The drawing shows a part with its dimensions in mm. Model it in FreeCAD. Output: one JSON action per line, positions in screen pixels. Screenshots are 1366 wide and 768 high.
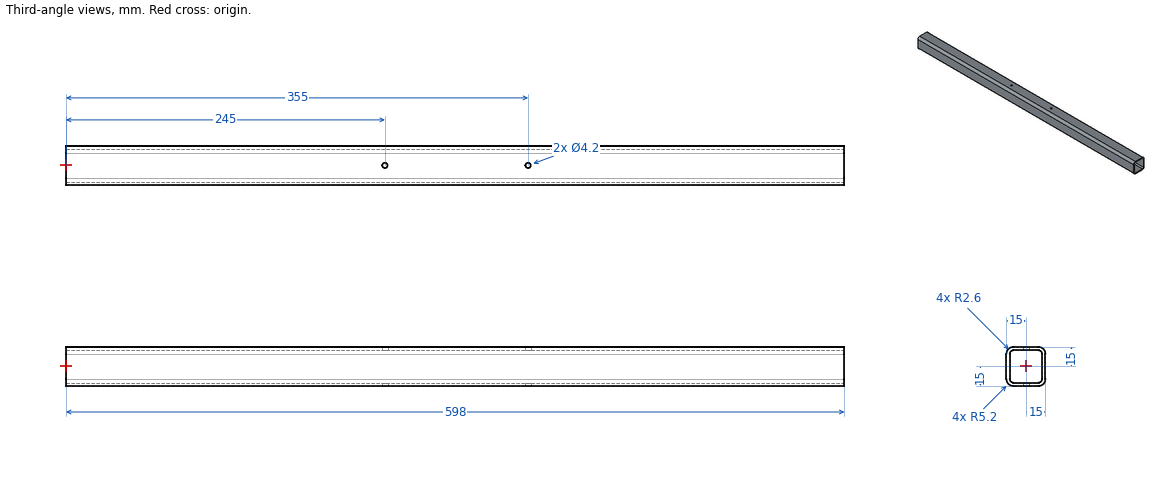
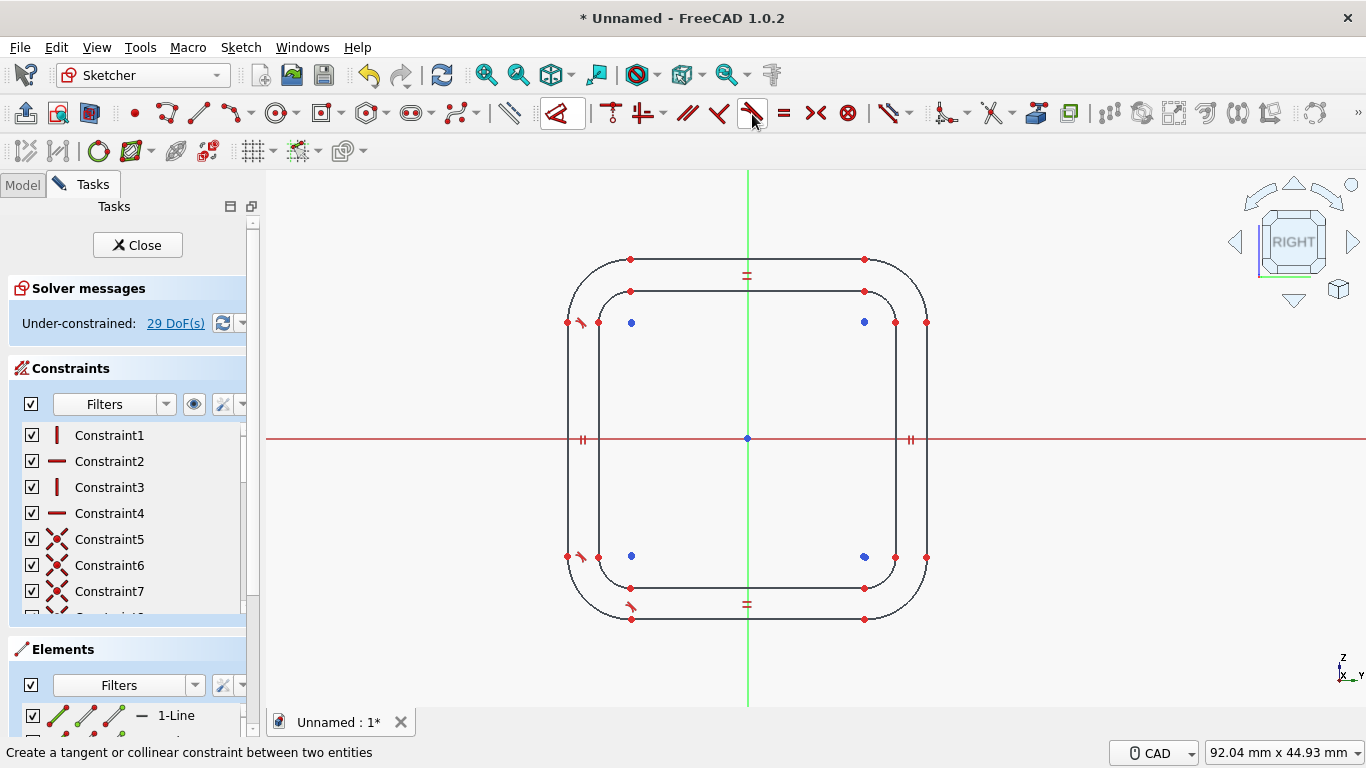
{"action": "left_click", "coordinate": [701, 619]}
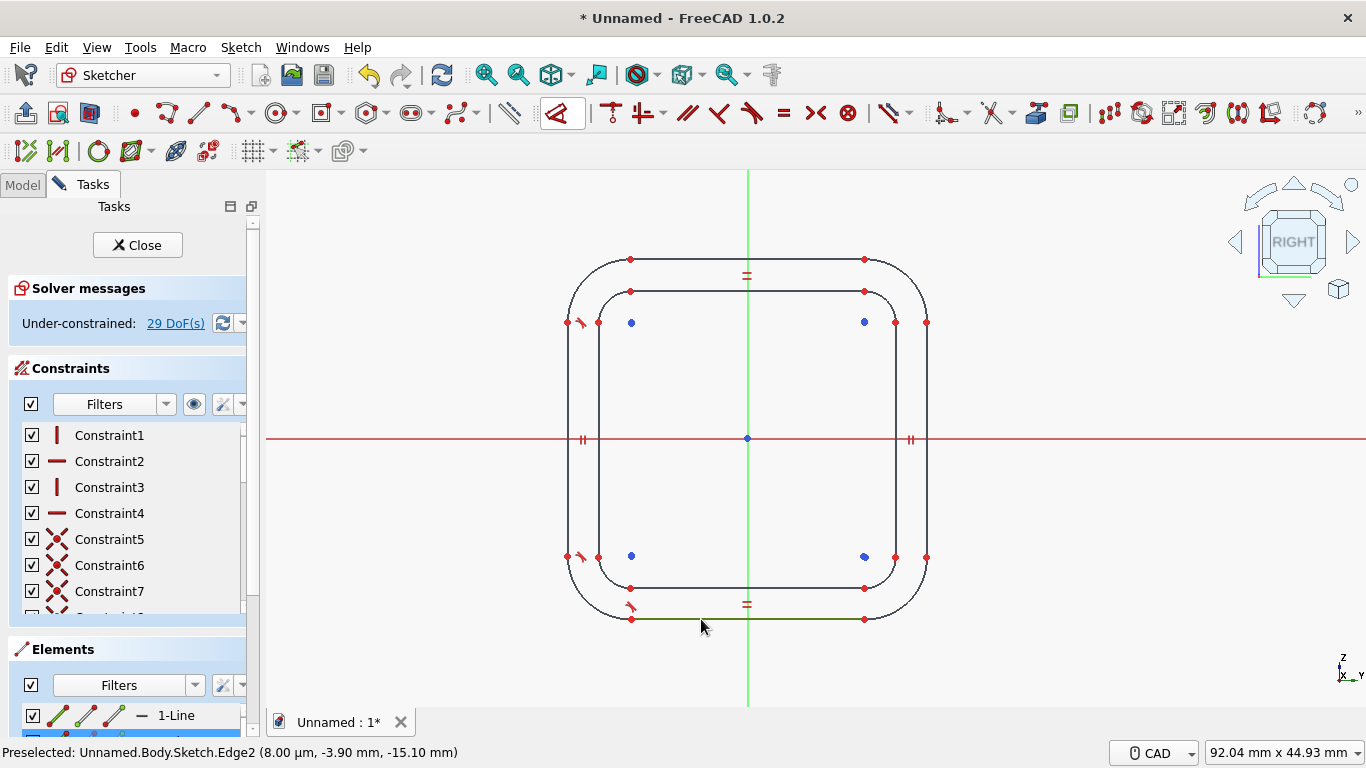
{"action": "left_click", "coordinate": [893, 613]}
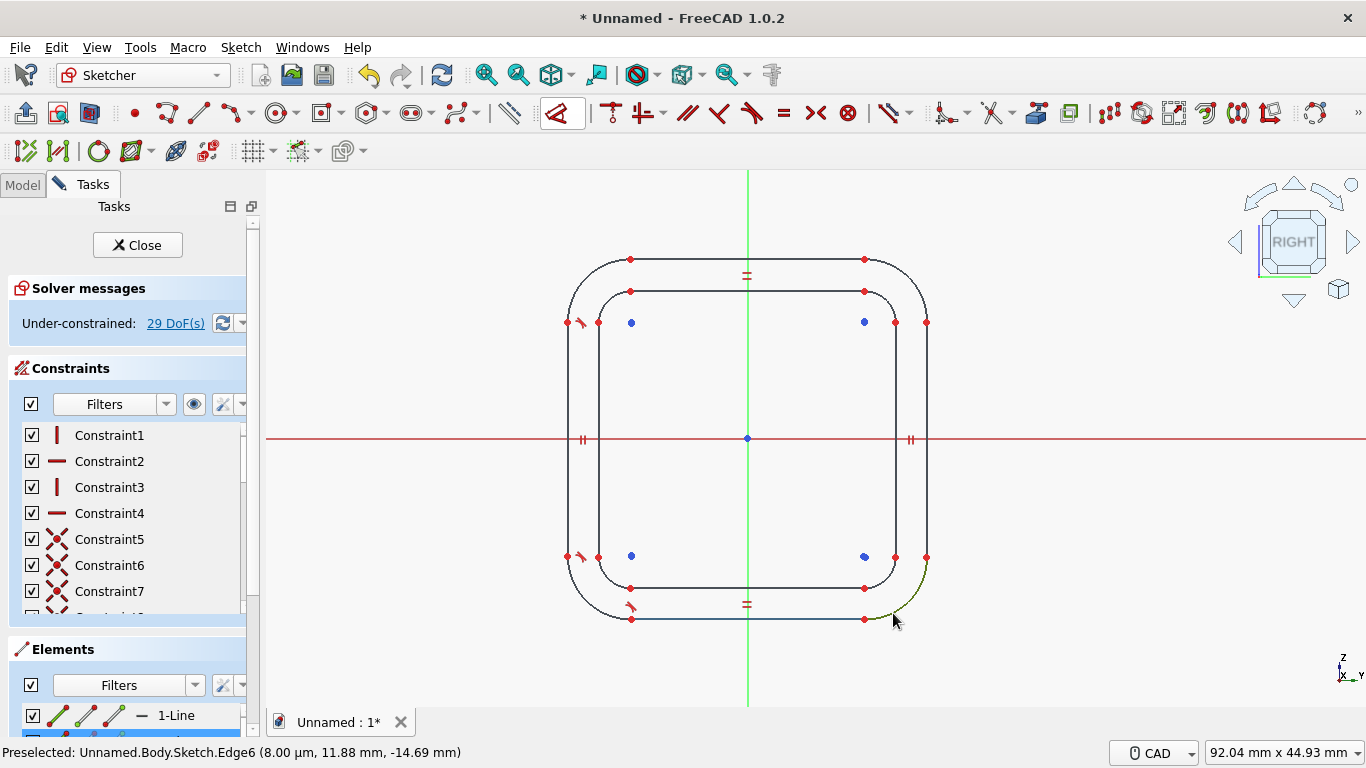
{"action": "left_click", "coordinate": [752, 114]}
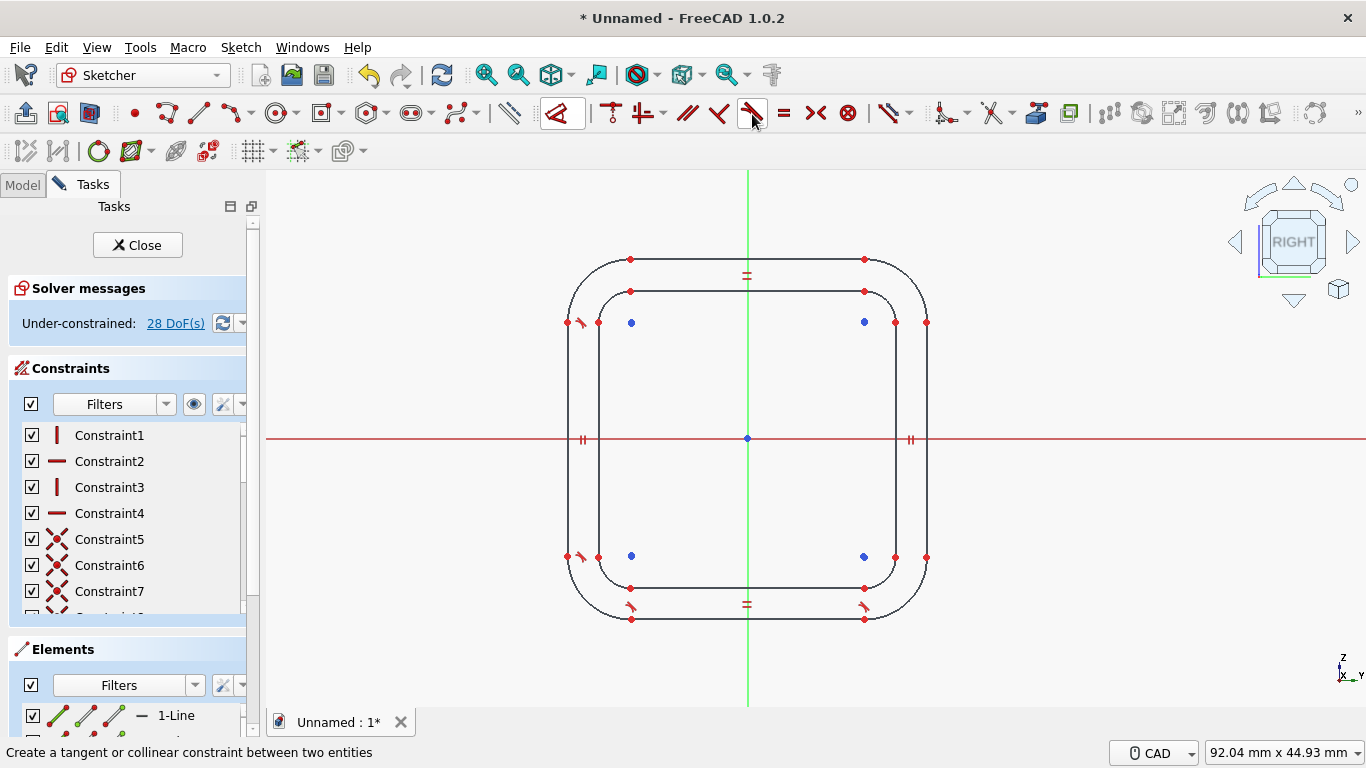
{"action": "left_click", "coordinate": [927, 487]}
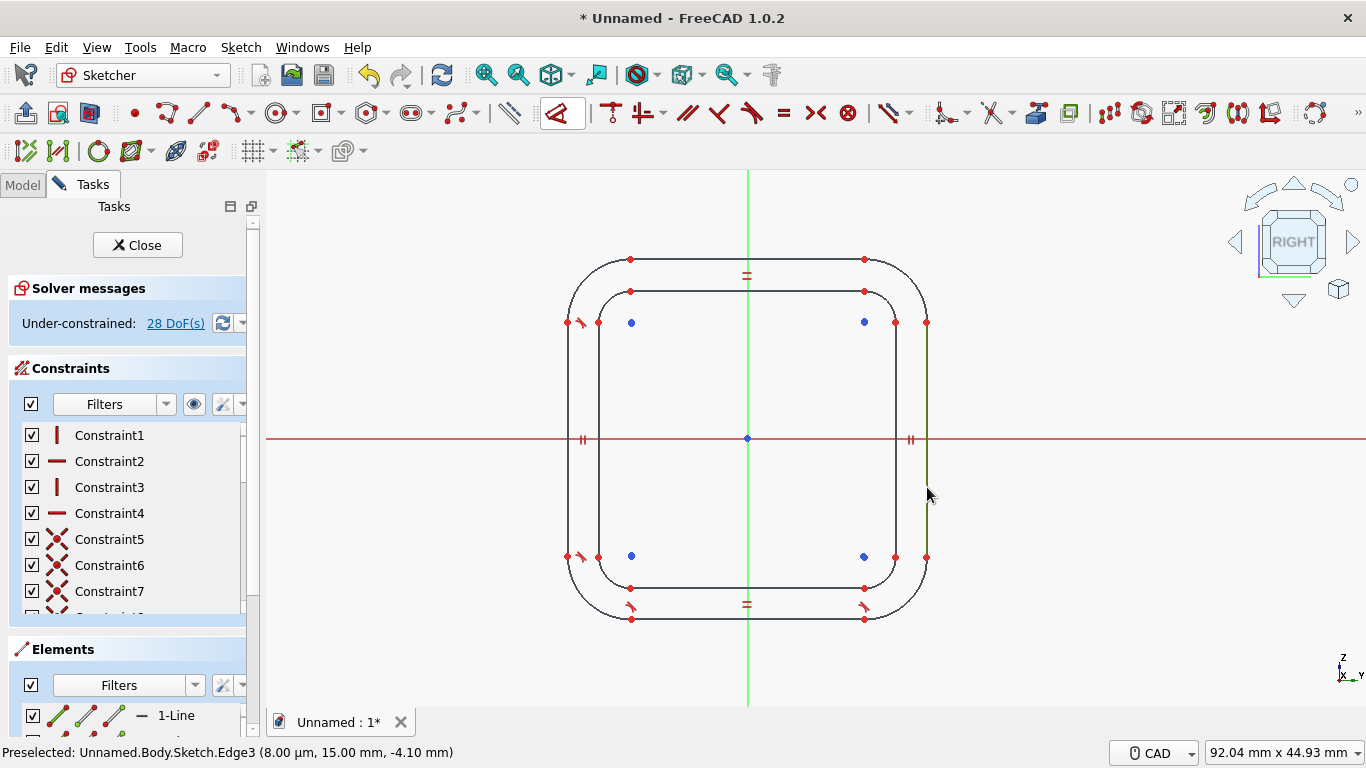
{"action": "left_click", "coordinate": [893, 613]}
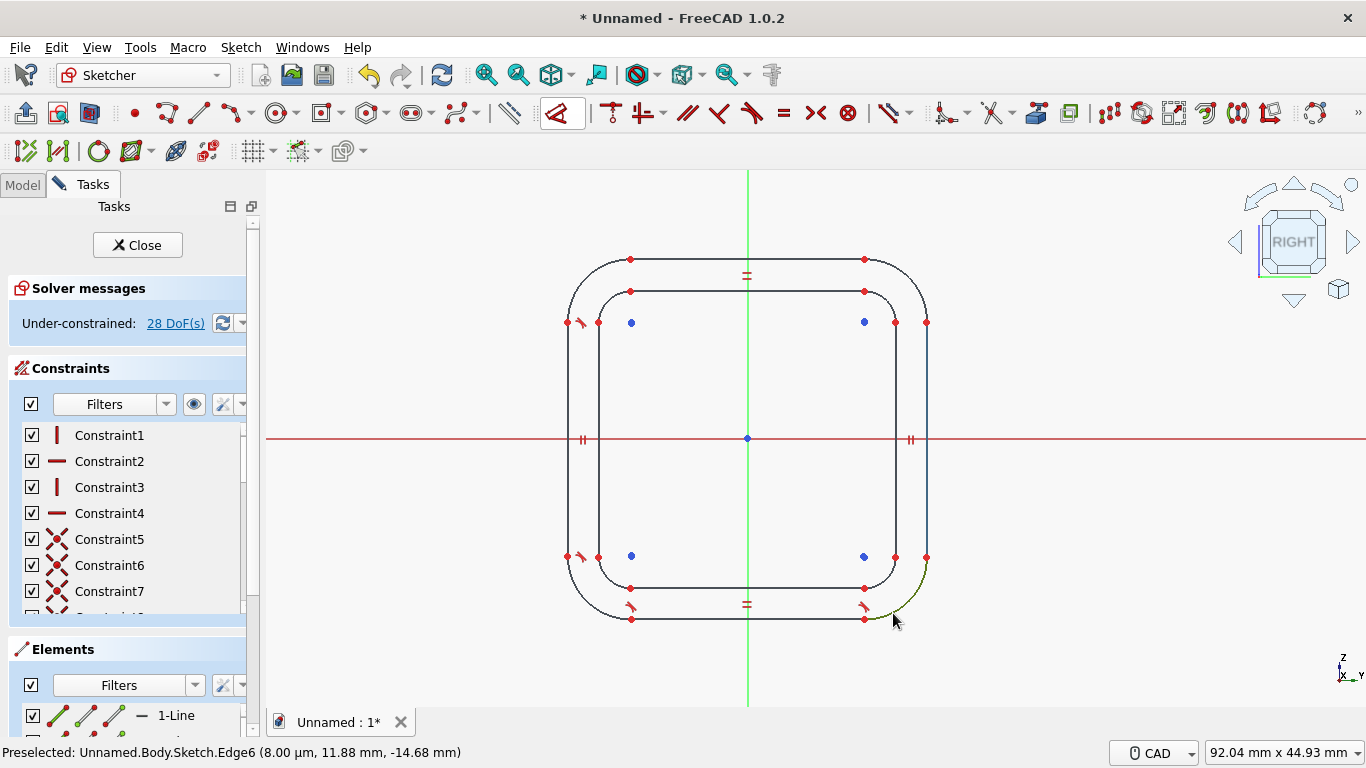
{"action": "key", "text": "t"}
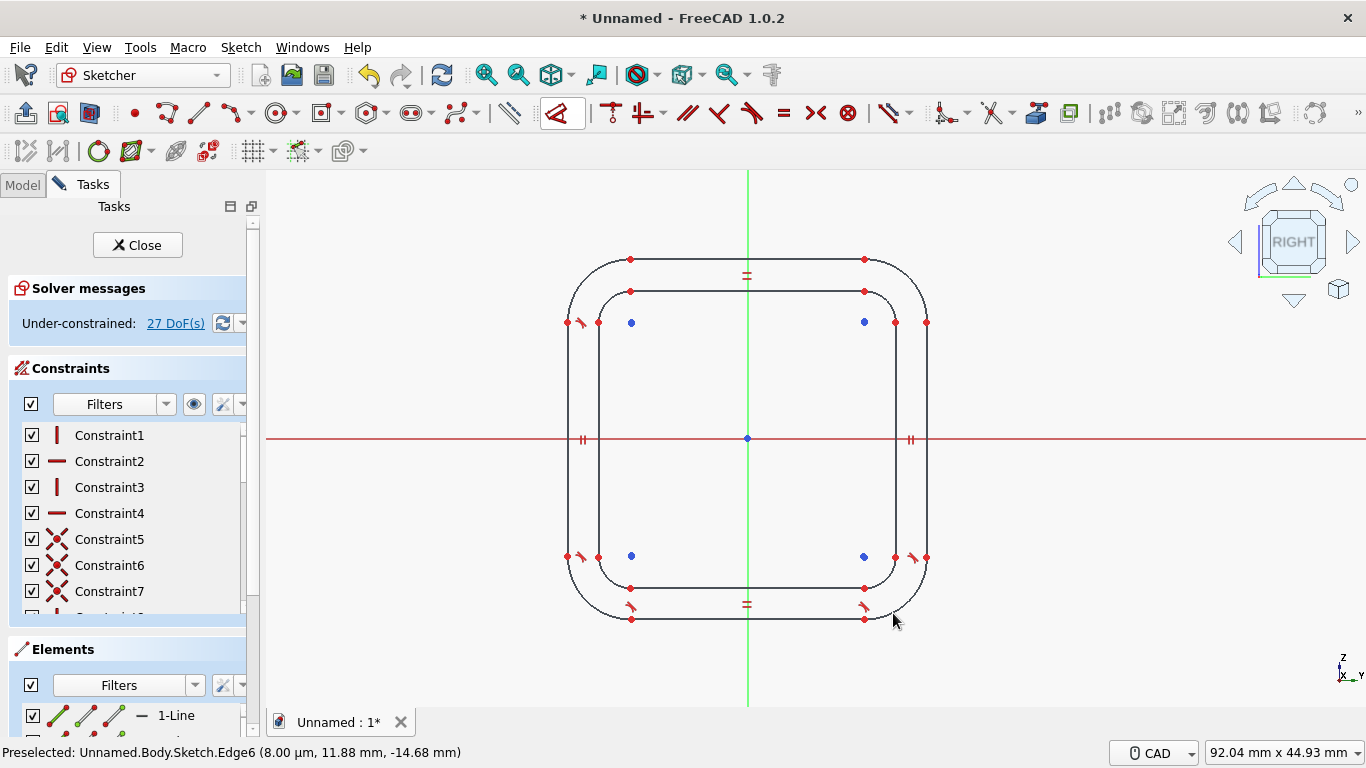
{"action": "left_click", "coordinate": [927, 487]}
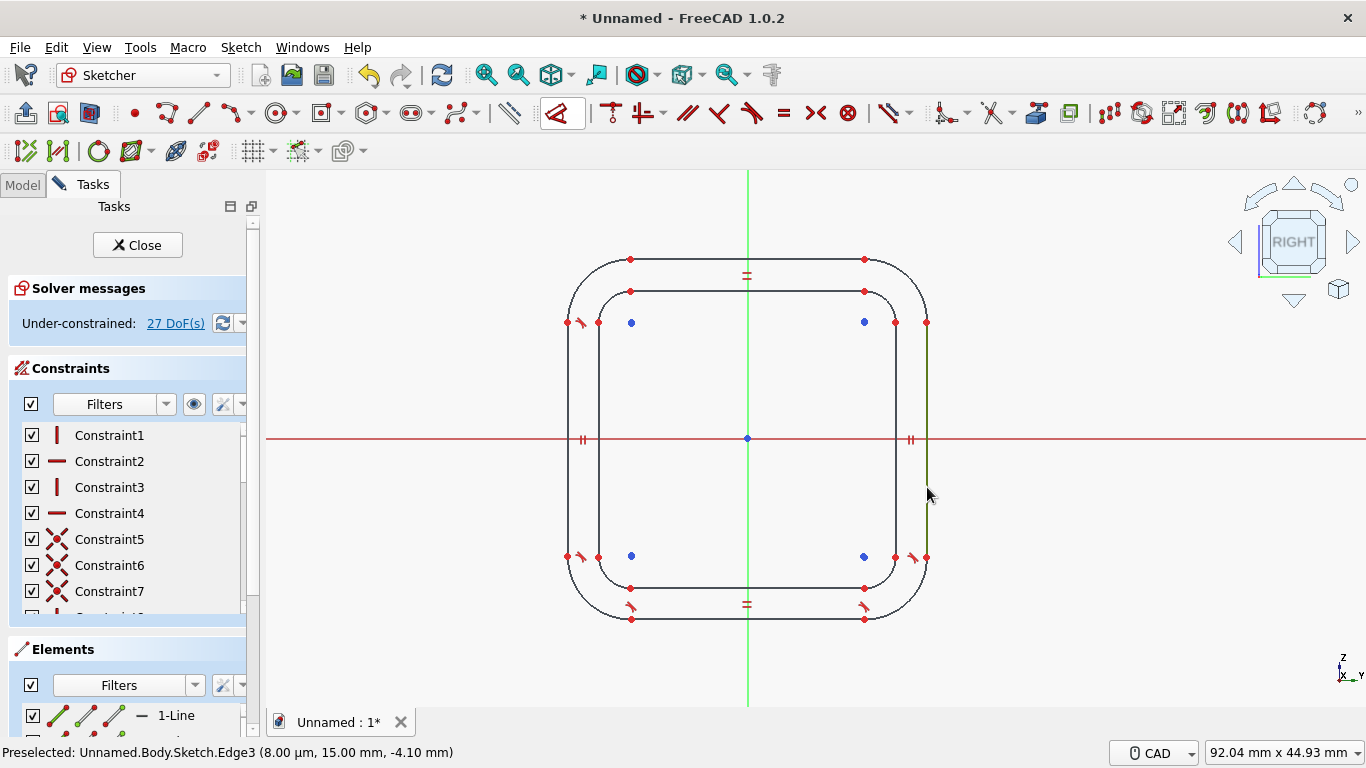
{"action": "left_click", "coordinate": [920, 294]}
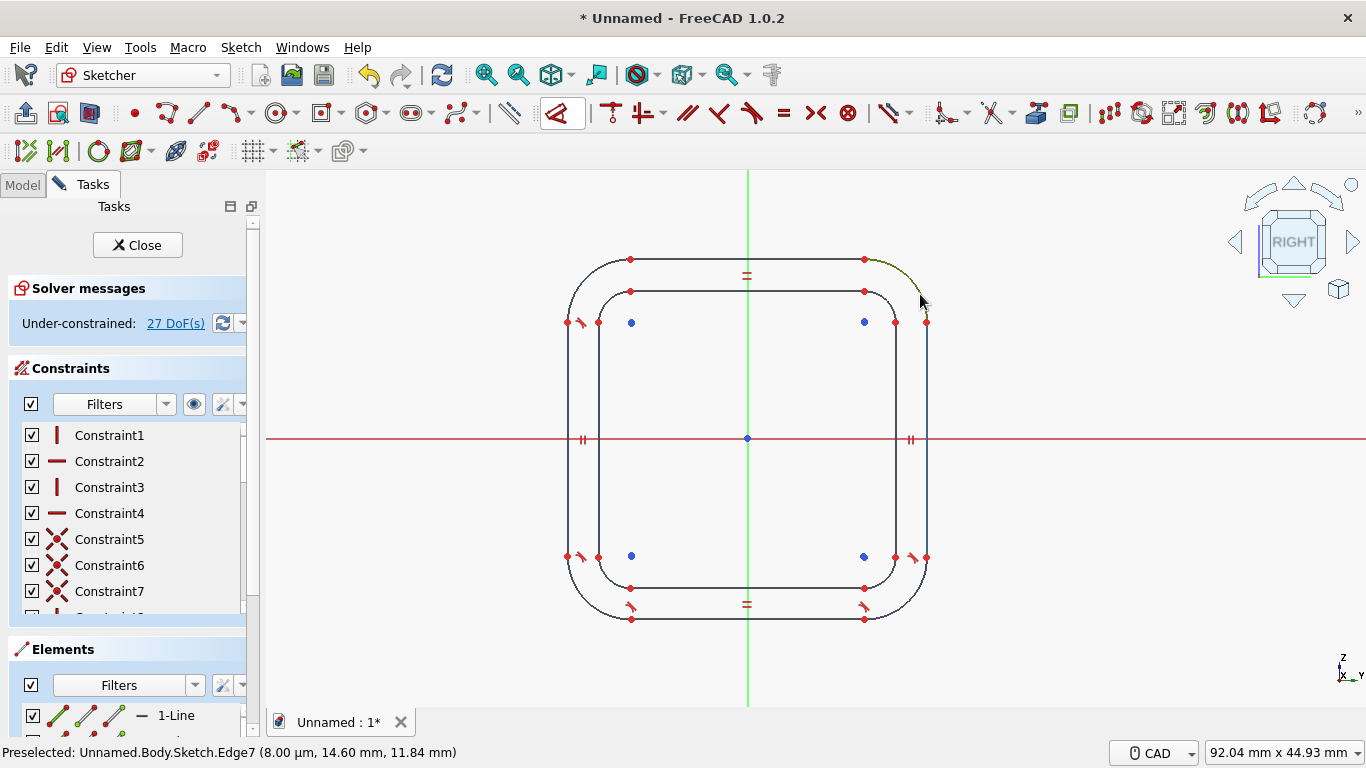
{"action": "key", "text": "t"}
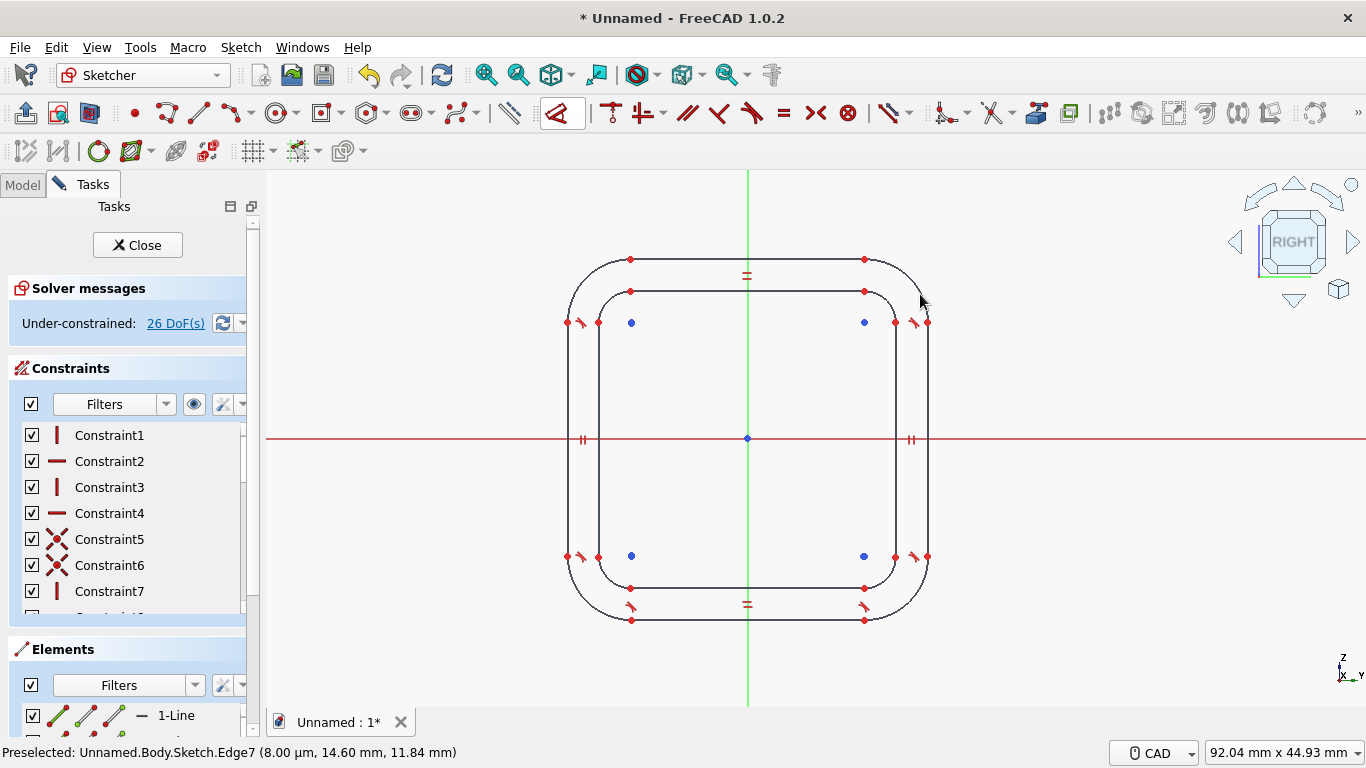
{"action": "left_click", "coordinate": [795, 259]}